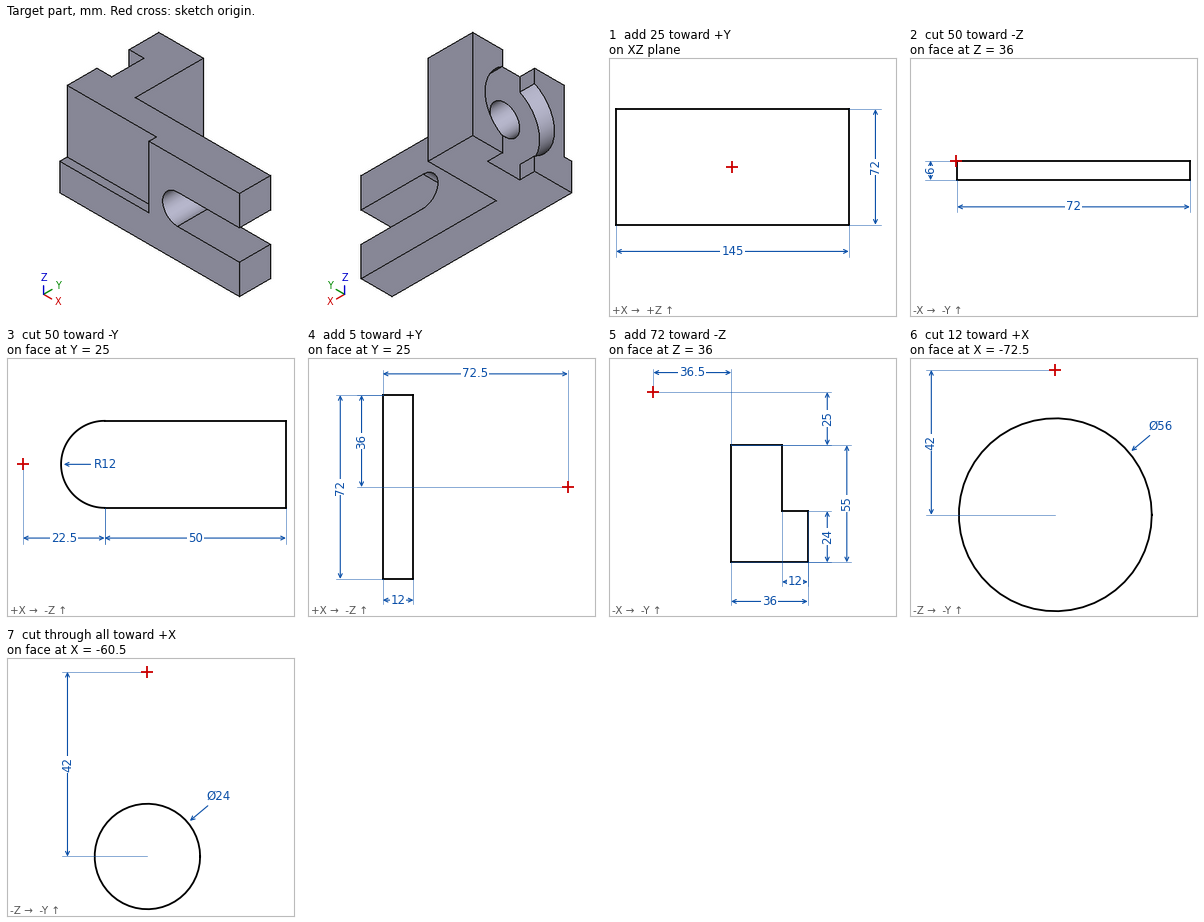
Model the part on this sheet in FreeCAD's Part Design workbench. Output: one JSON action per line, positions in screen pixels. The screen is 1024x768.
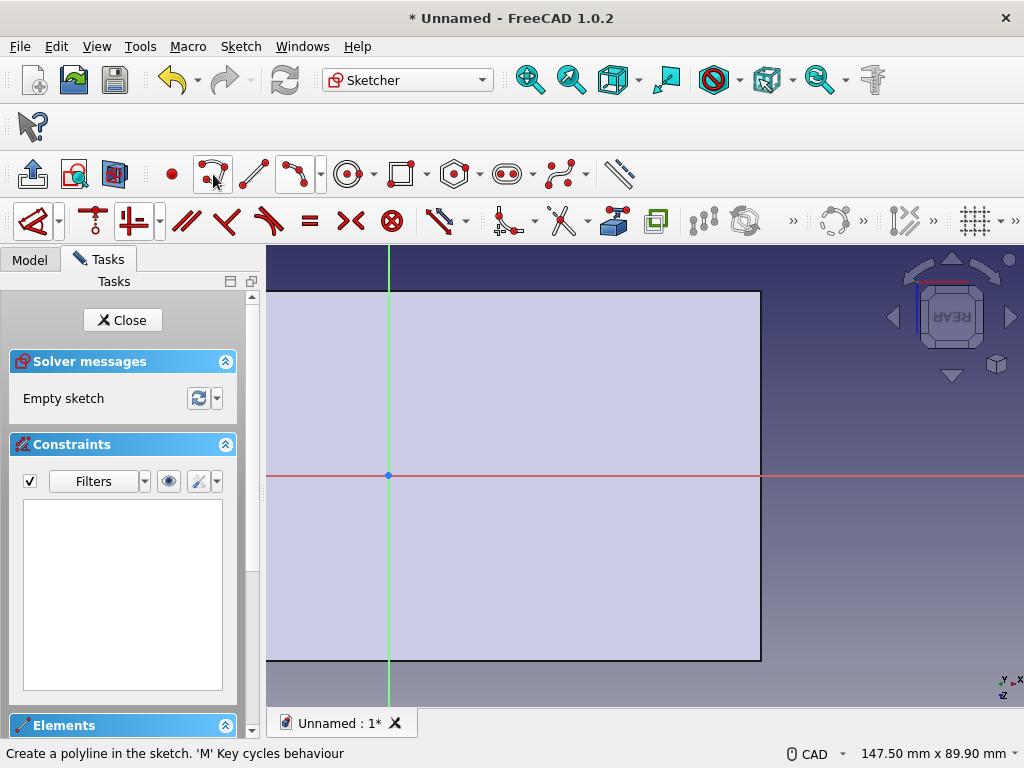
{"action": "left_click", "coordinate": [504, 537]}
{"action": "left_click", "coordinate": [761, 537]}
{"action": "left_click", "coordinate": [761, 414]}
{"action": "left_click", "coordinate": [504, 414]}
{"action": "right_click", "coordinate": [504, 414]}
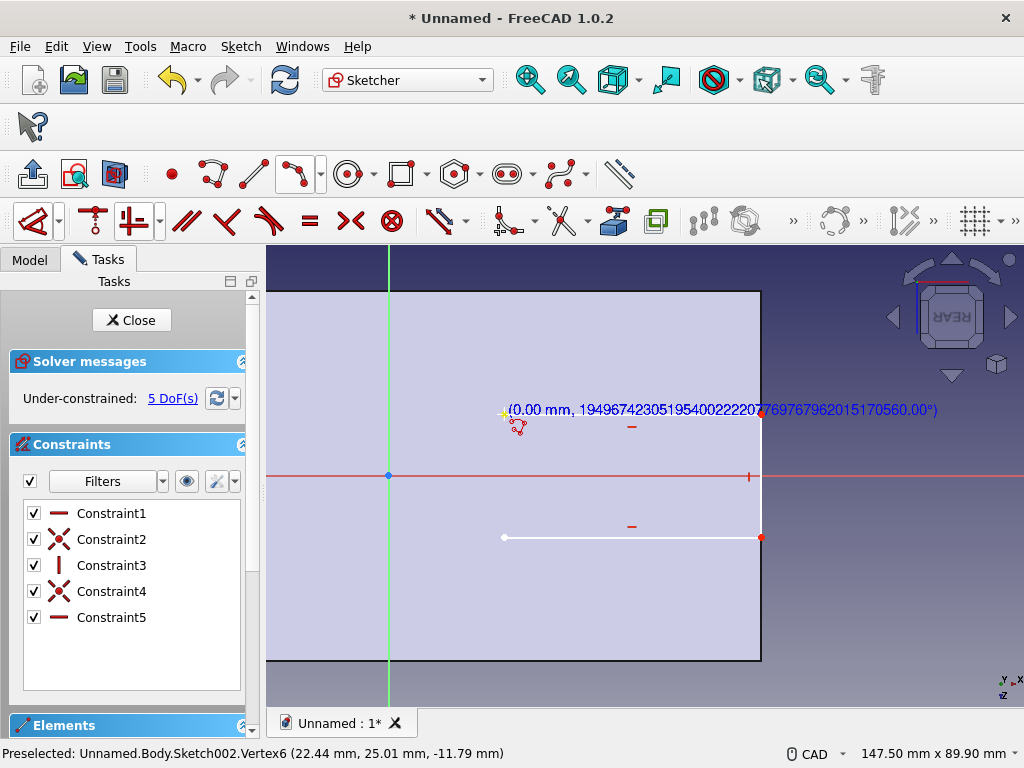
{"action": "left_click", "coordinate": [294, 174]}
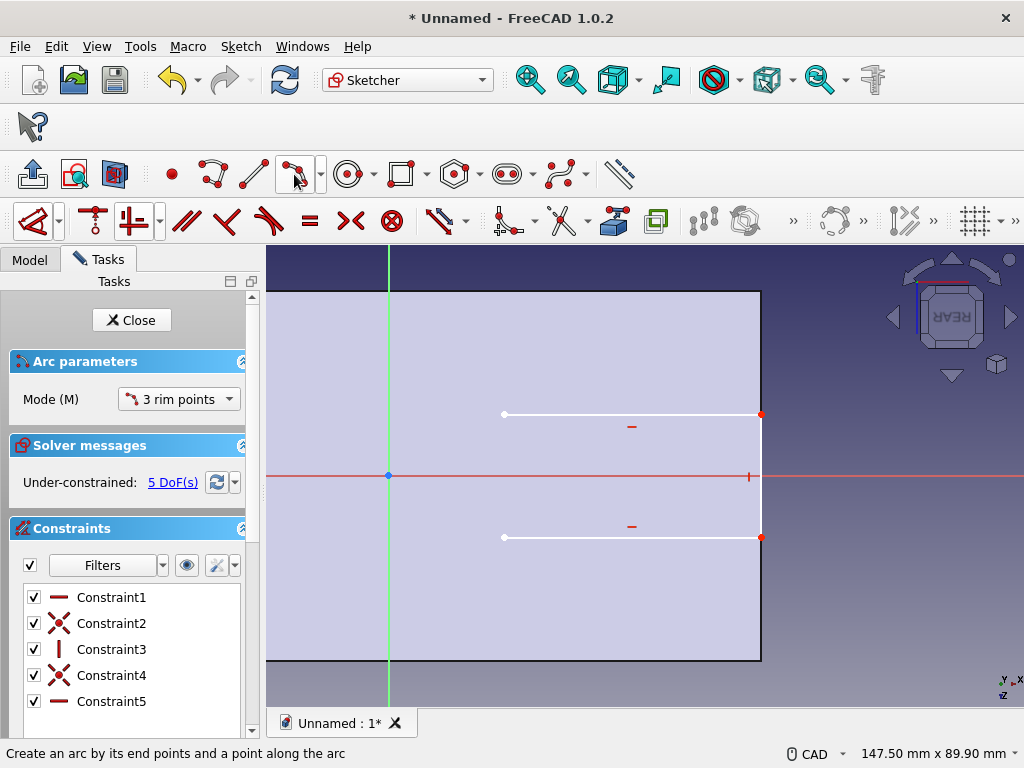
{"action": "left_click", "coordinate": [504, 415]}
{"action": "left_click", "coordinate": [504, 538]}
{"action": "left_click", "coordinate": [446, 457]}
{"action": "key", "text": "Escape"}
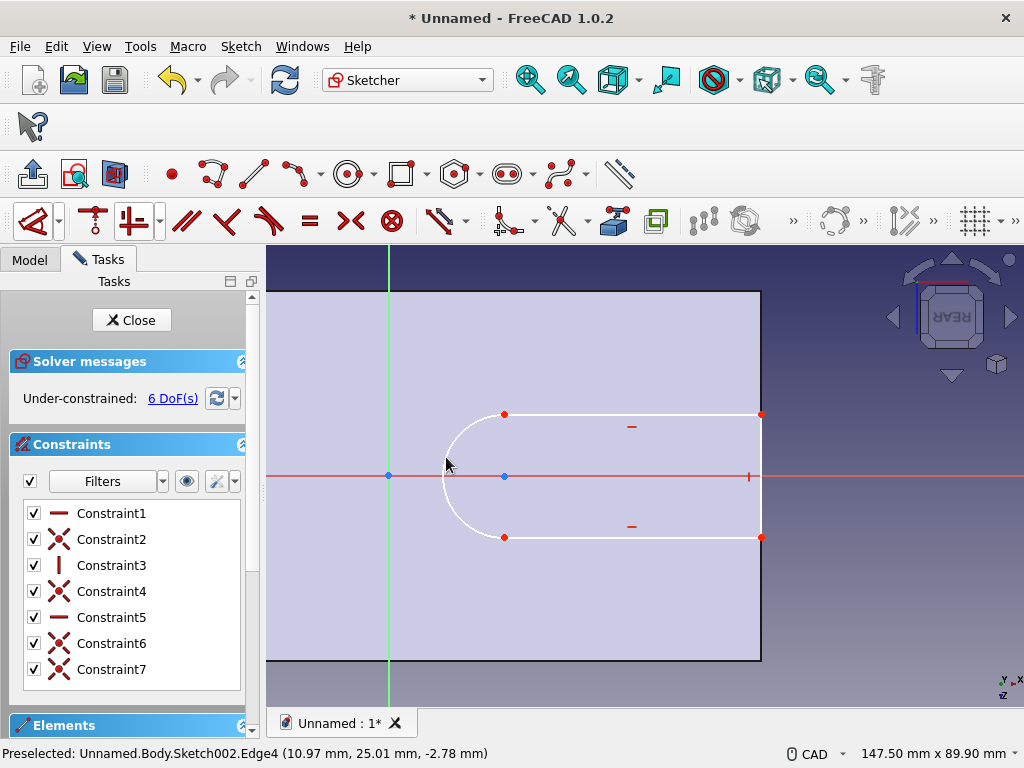
{"action": "left_click", "coordinate": [581, 538]}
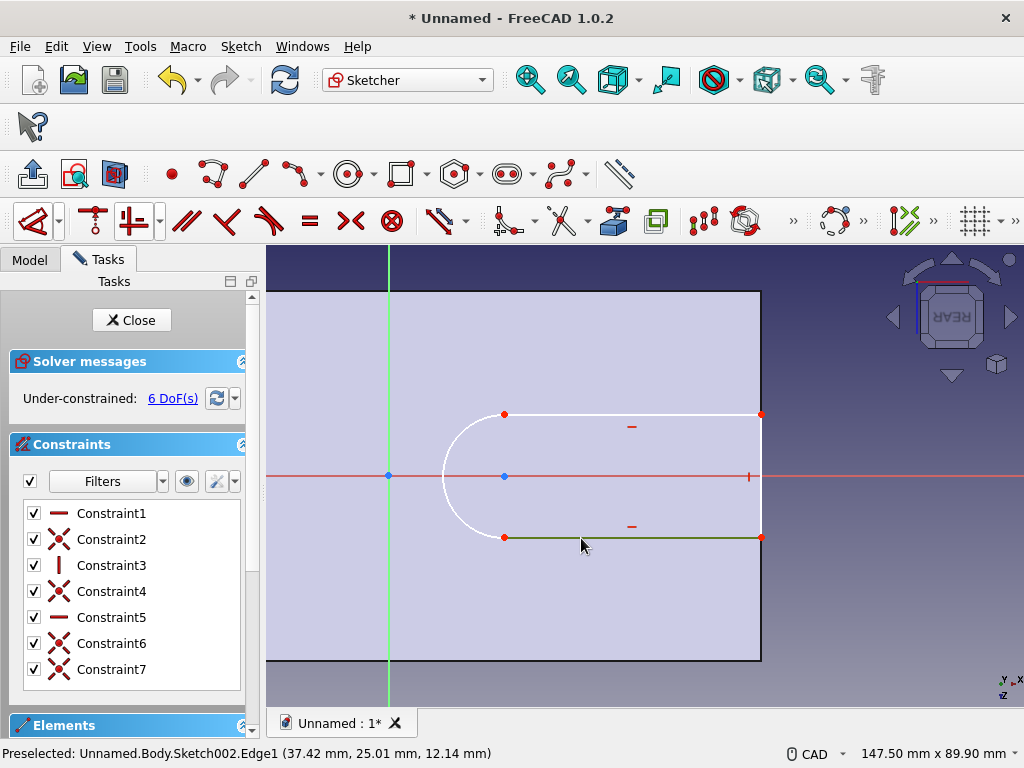
{"action": "left_click", "coordinate": [455, 441]}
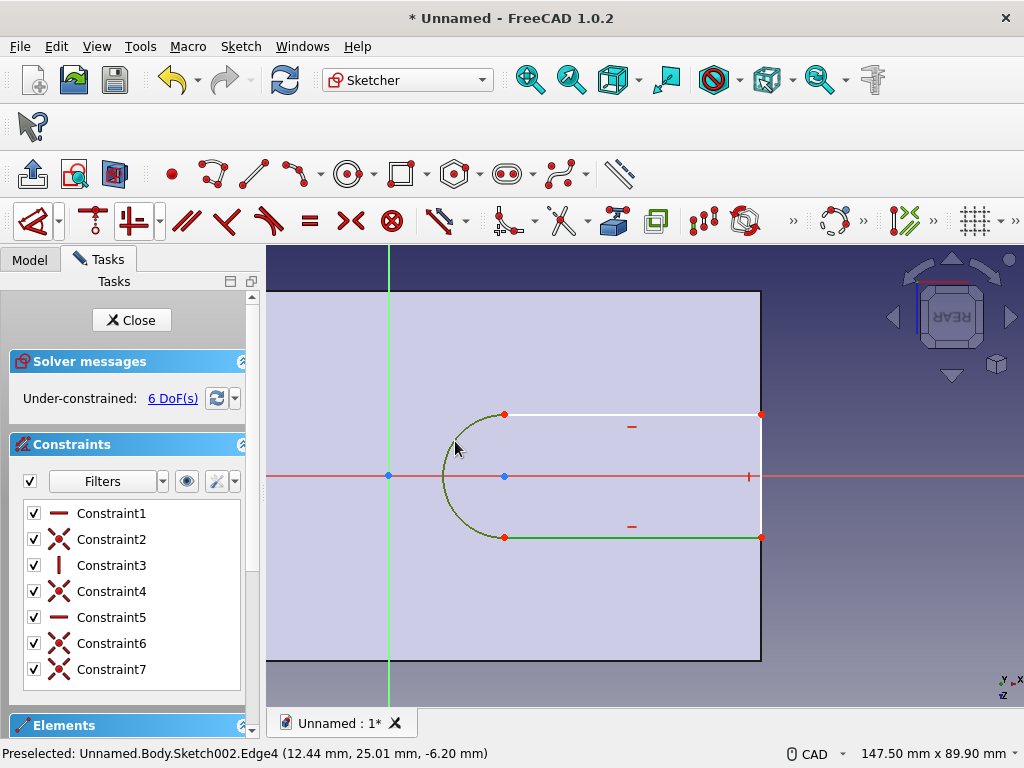
{"action": "left_click", "coordinate": [269, 222]}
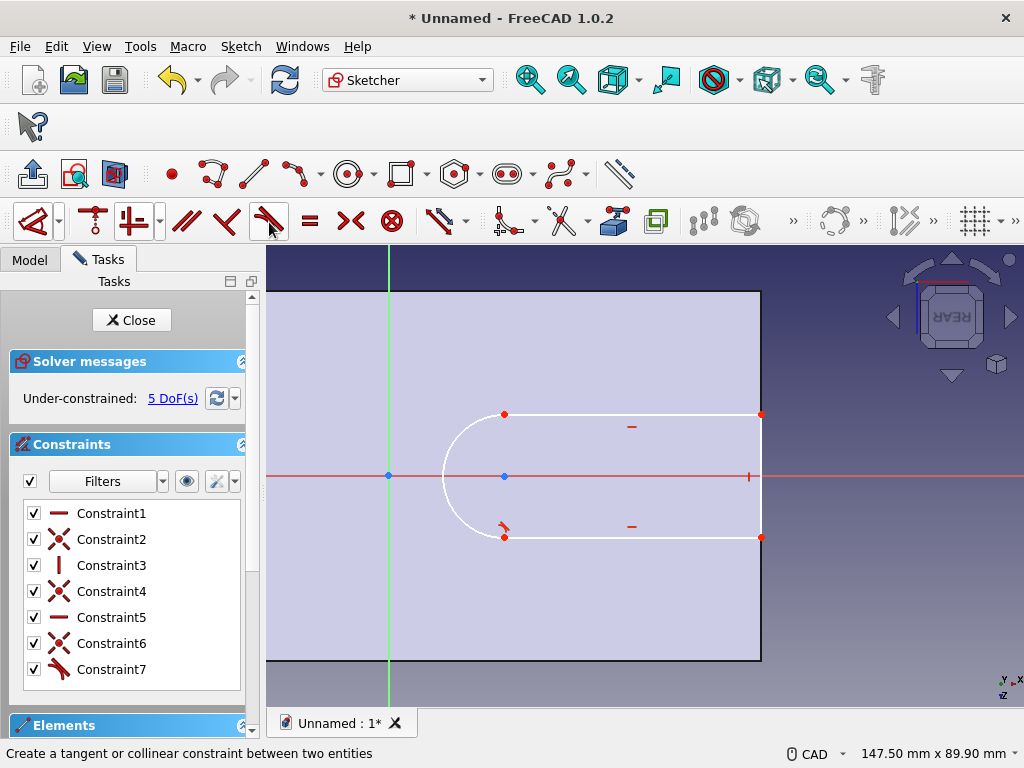
{"action": "left_click", "coordinate": [684, 415]}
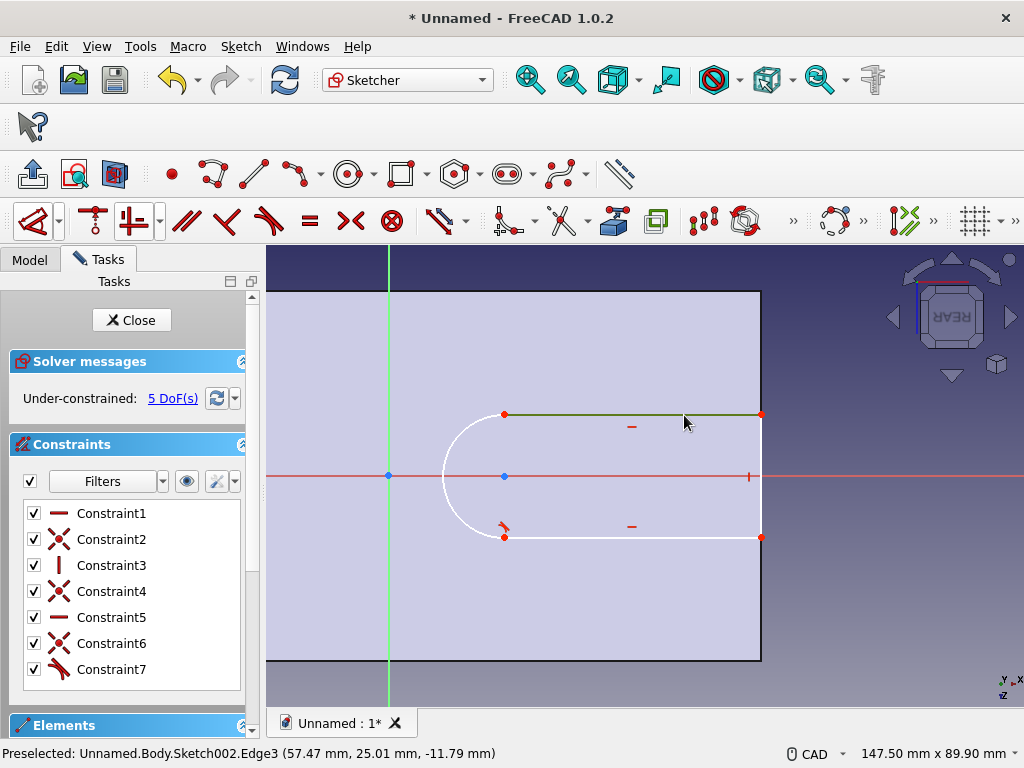
{"action": "left_click", "coordinate": [455, 441]}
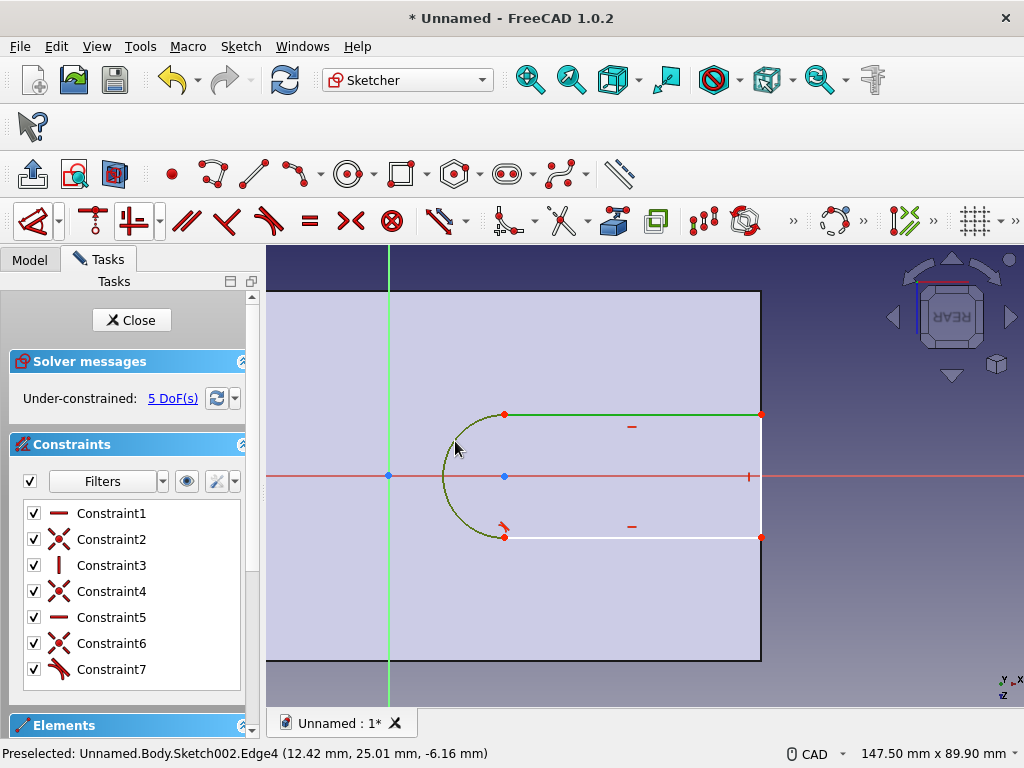
{"action": "left_click", "coordinate": [269, 222]}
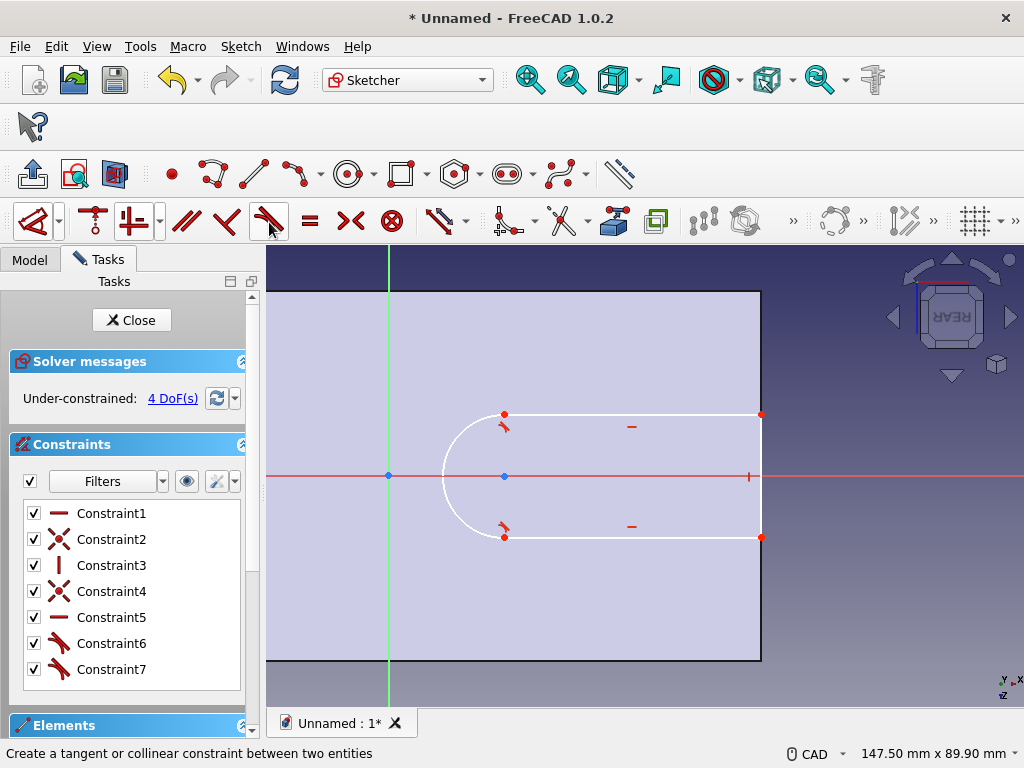
{"action": "left_click", "coordinate": [505, 476]}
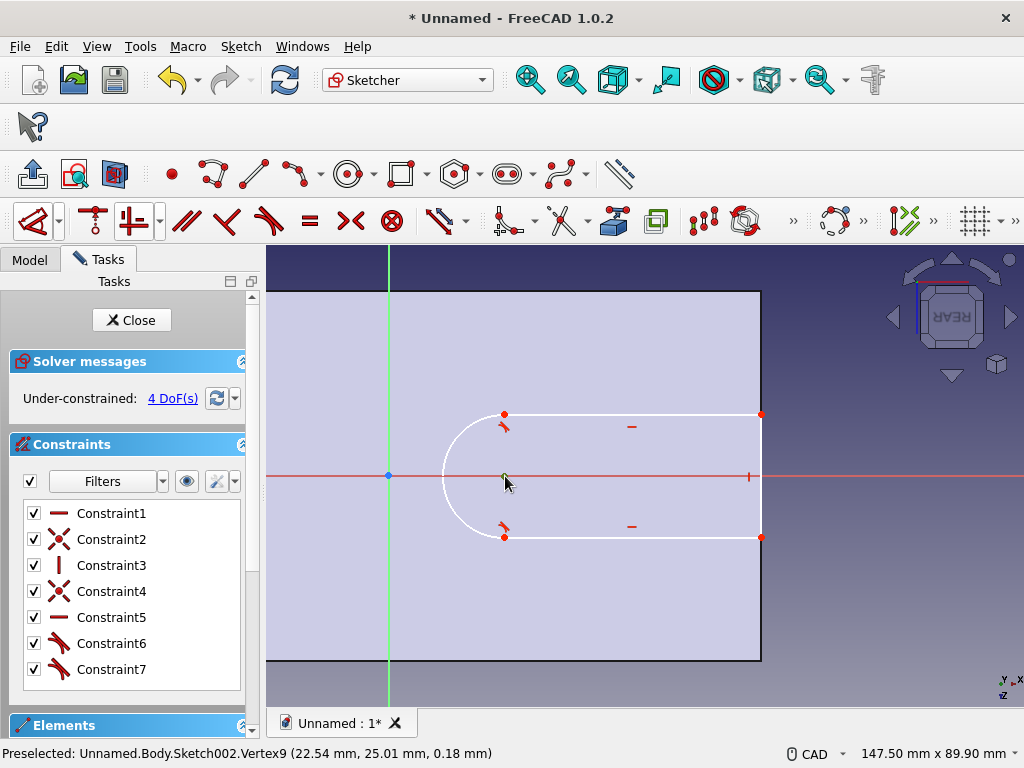
{"action": "left_click", "coordinate": [334, 476]}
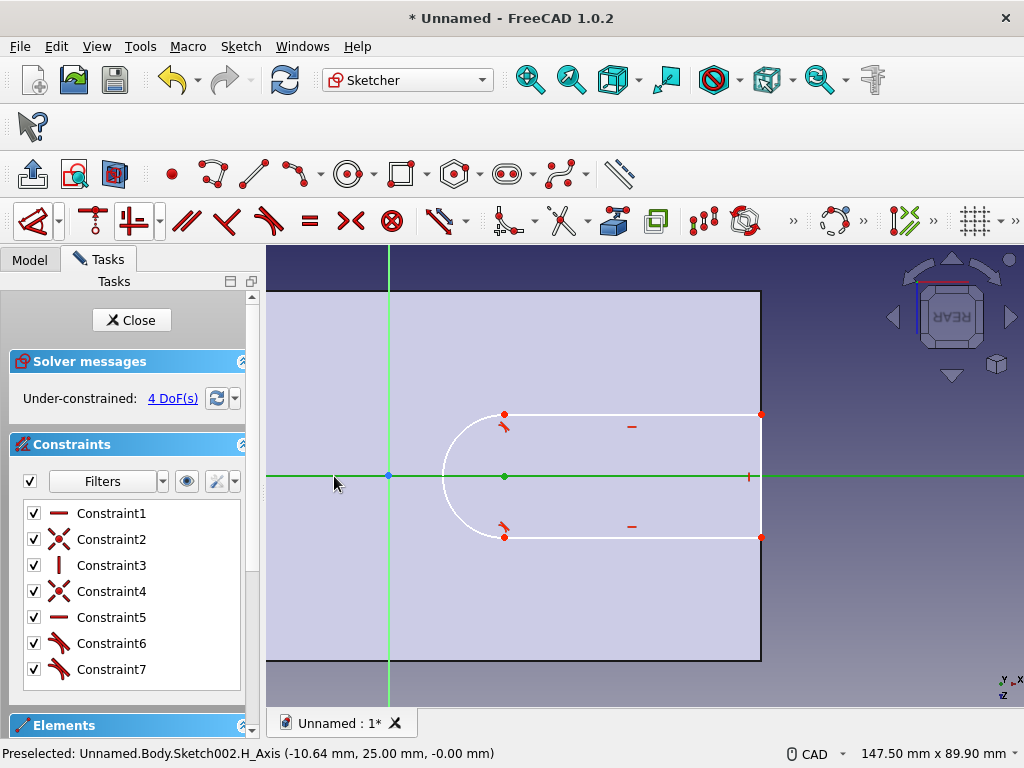
{"action": "left_click", "coordinate": [93, 222]}